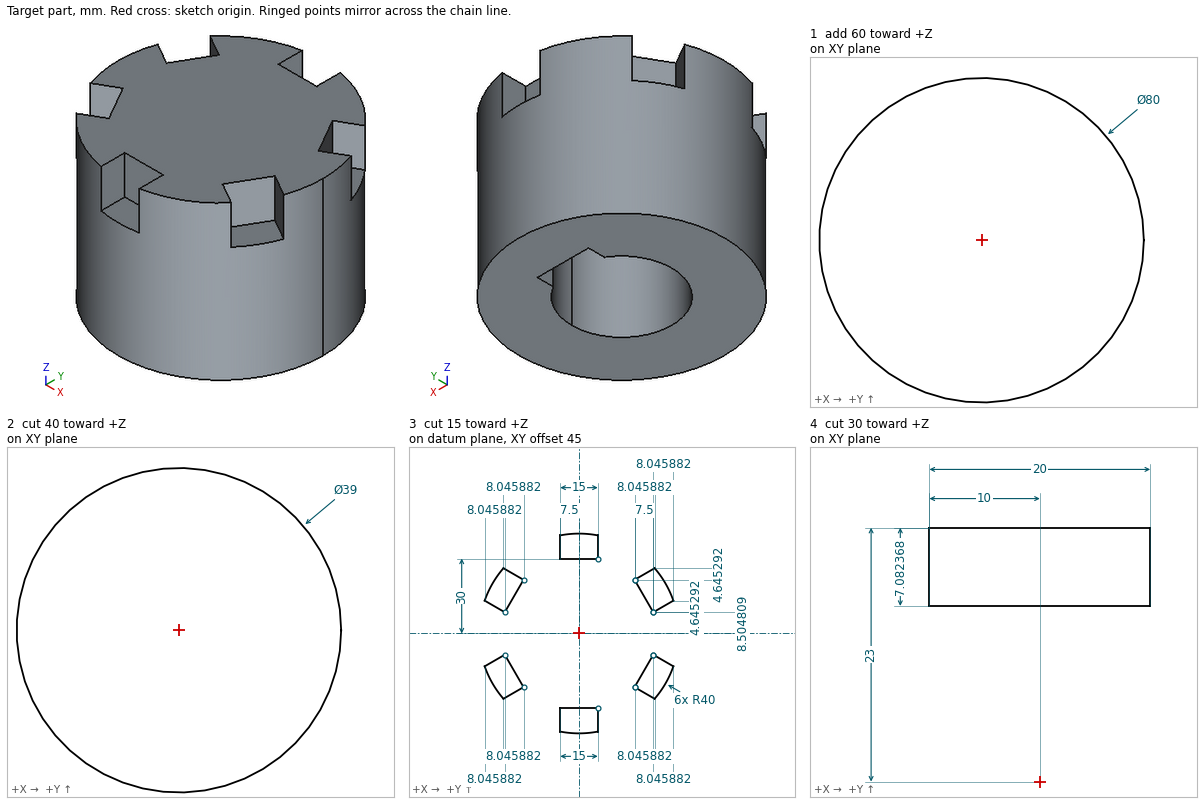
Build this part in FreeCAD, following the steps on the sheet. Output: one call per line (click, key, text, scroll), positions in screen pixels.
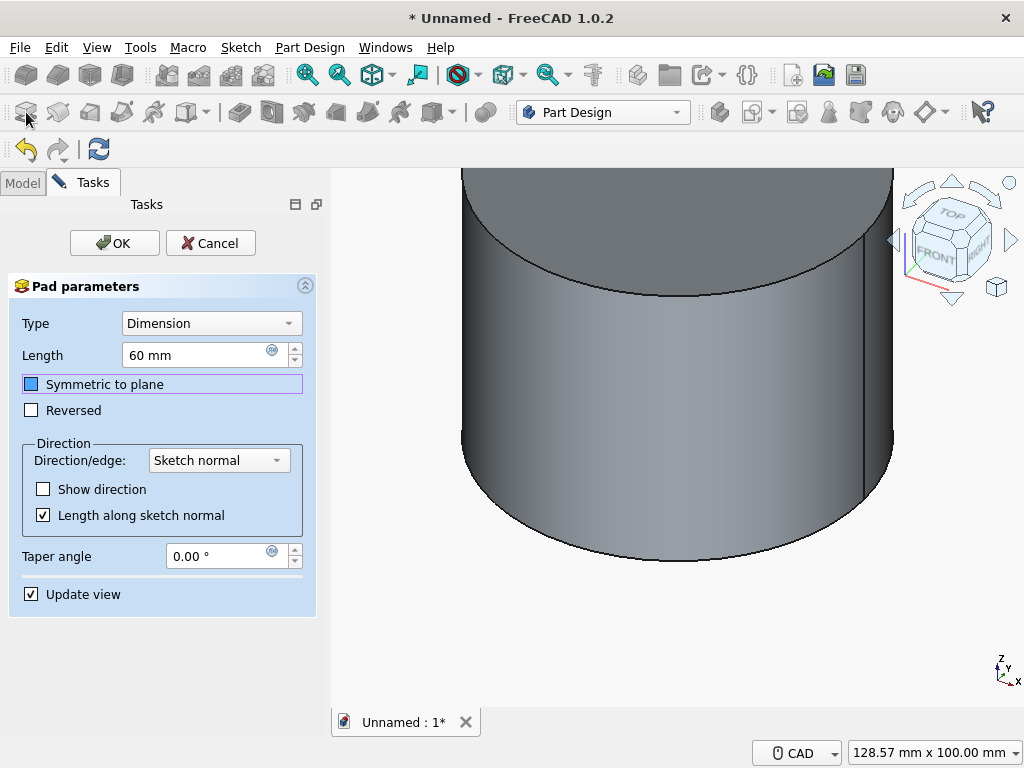
click(115, 243)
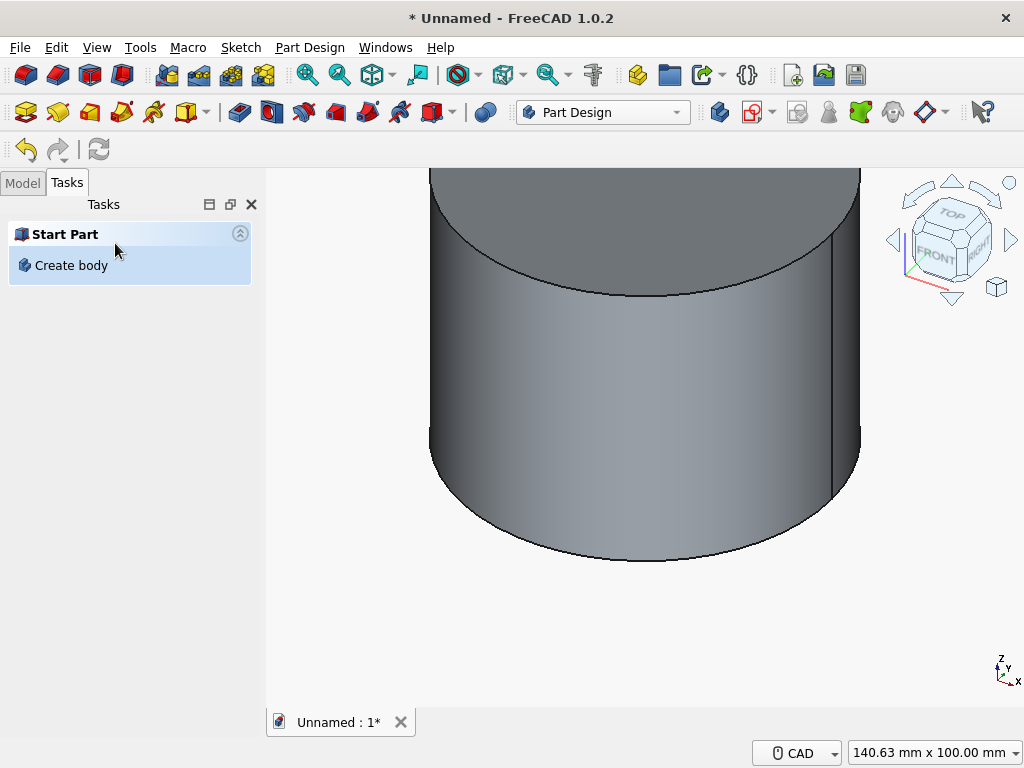
click(308, 76)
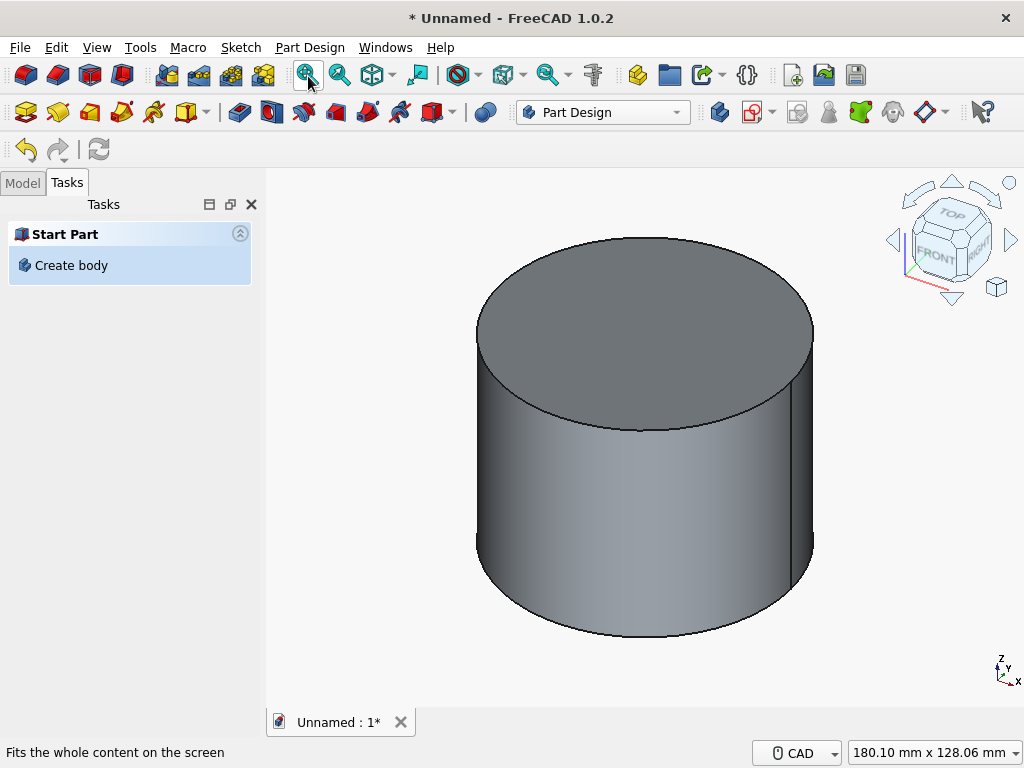
click(752, 112)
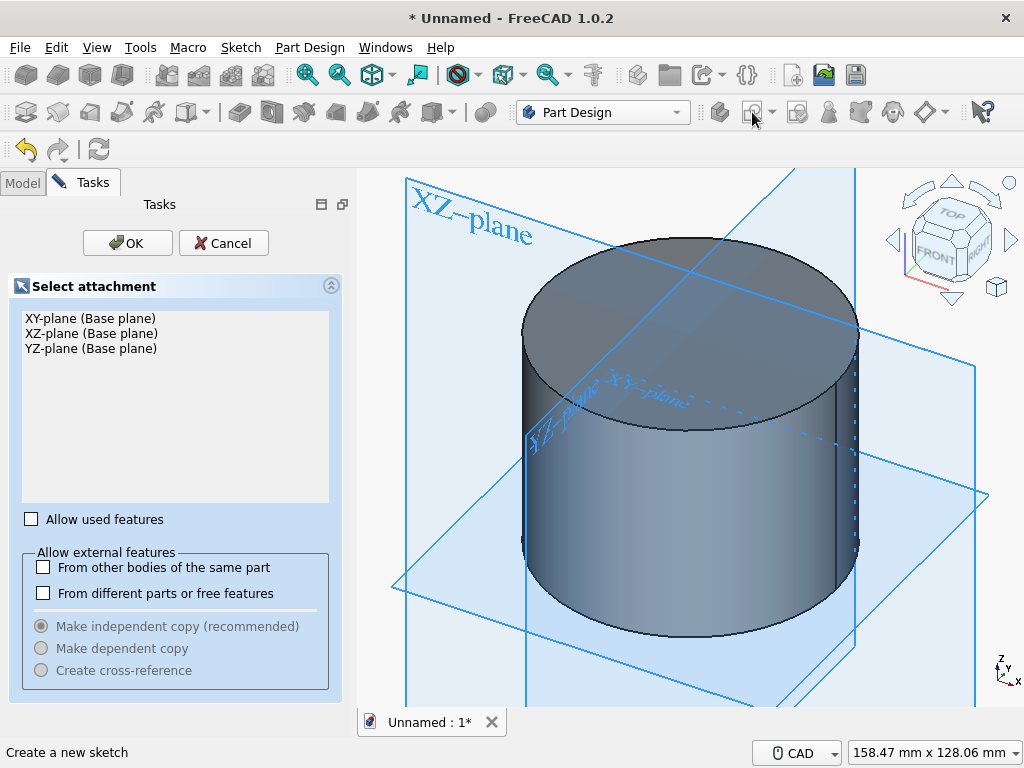
click(82, 318)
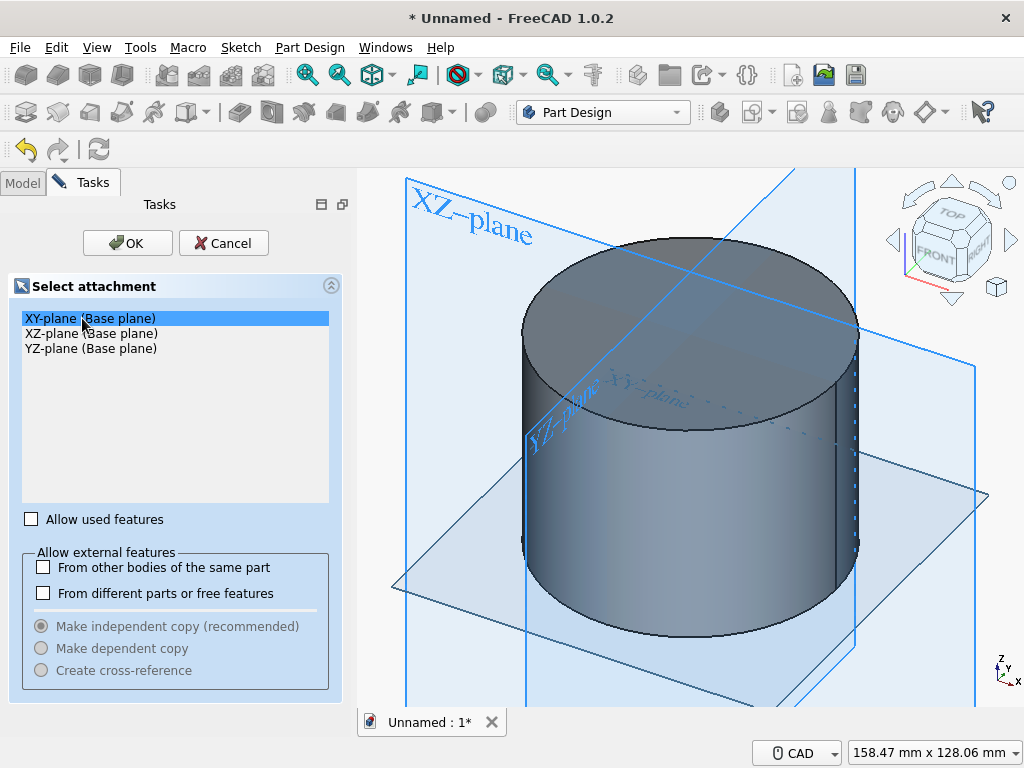
click(128, 243)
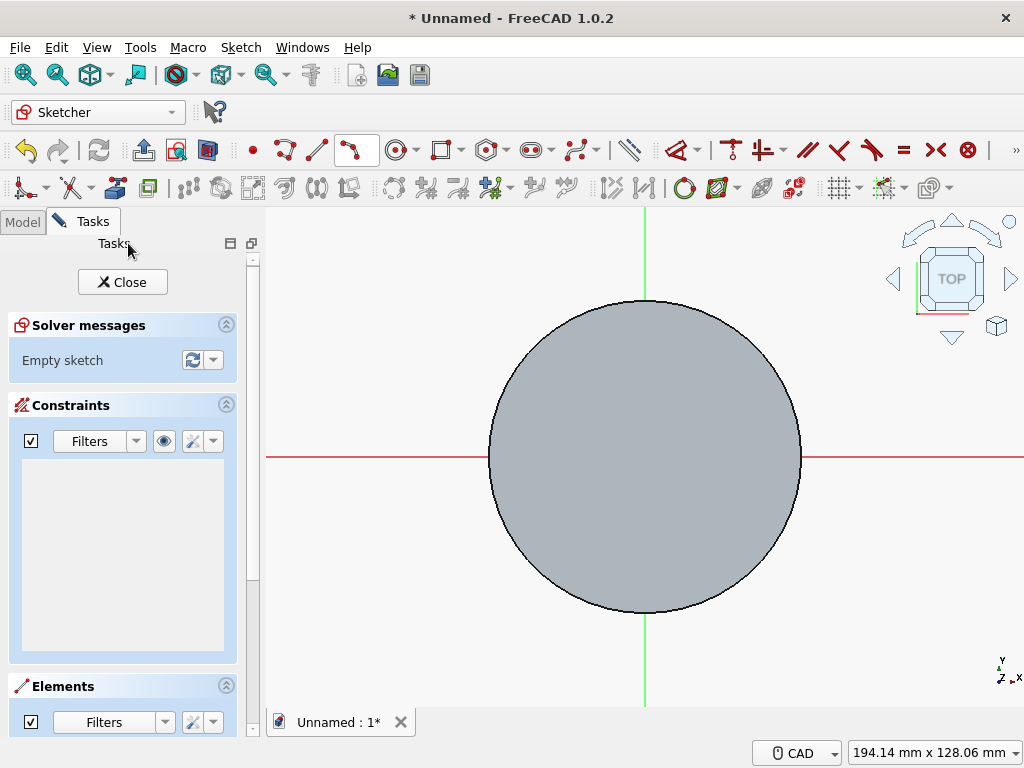
click(208, 150)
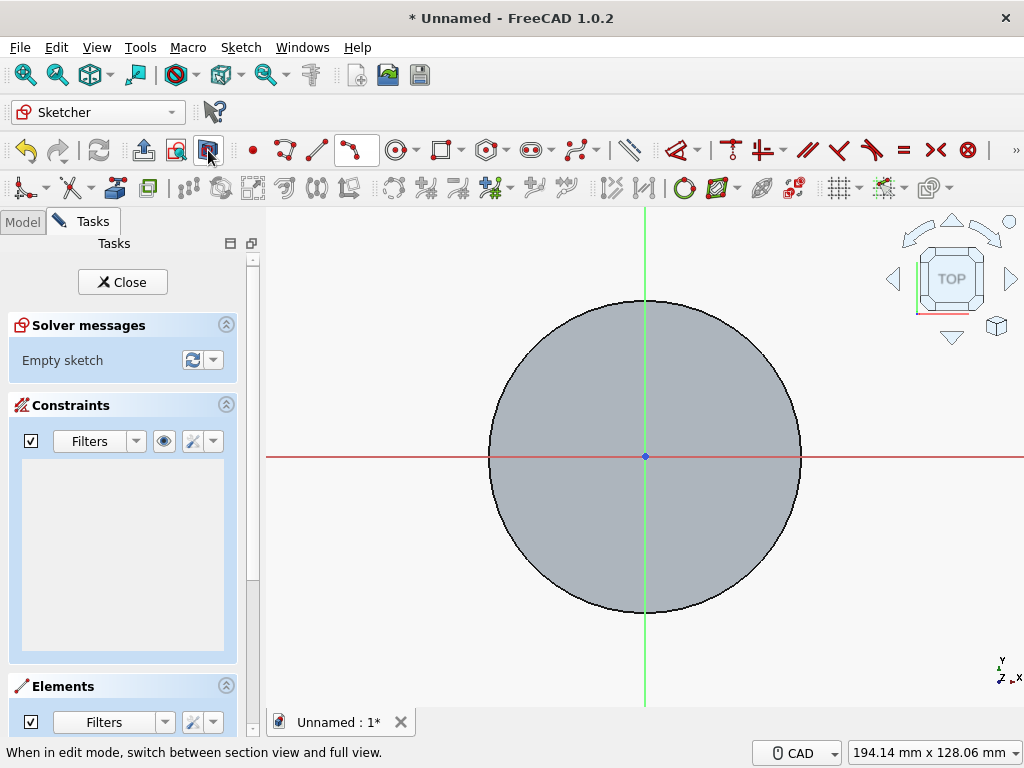
scroll(701, 457, up, 4)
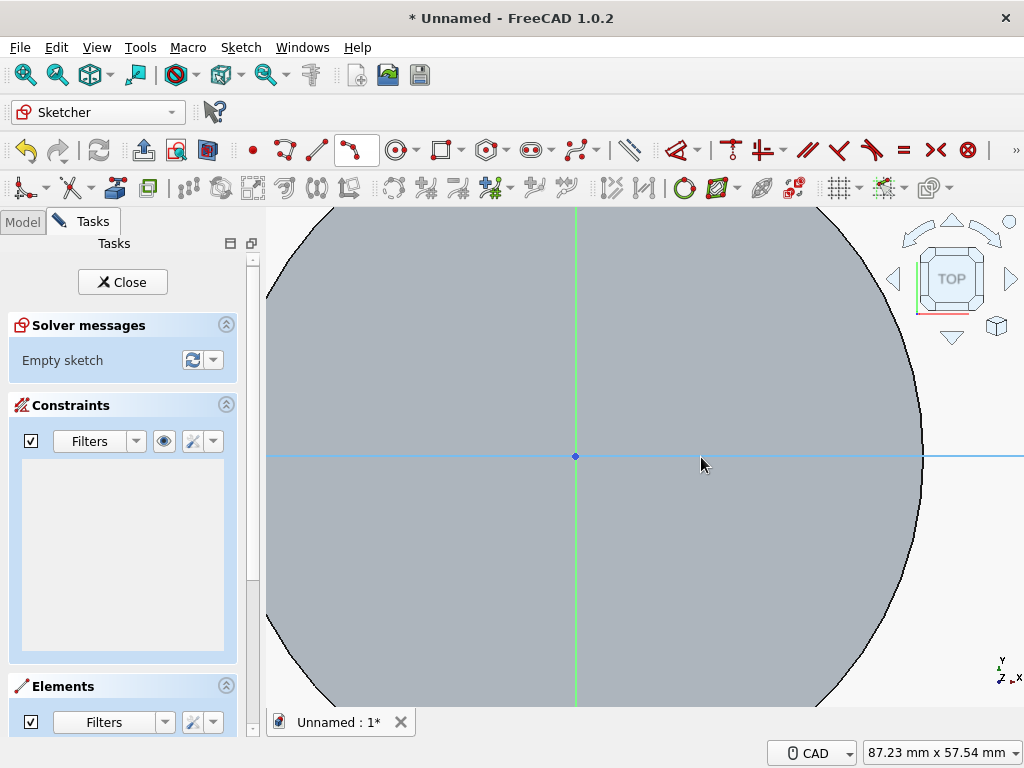
click(396, 150)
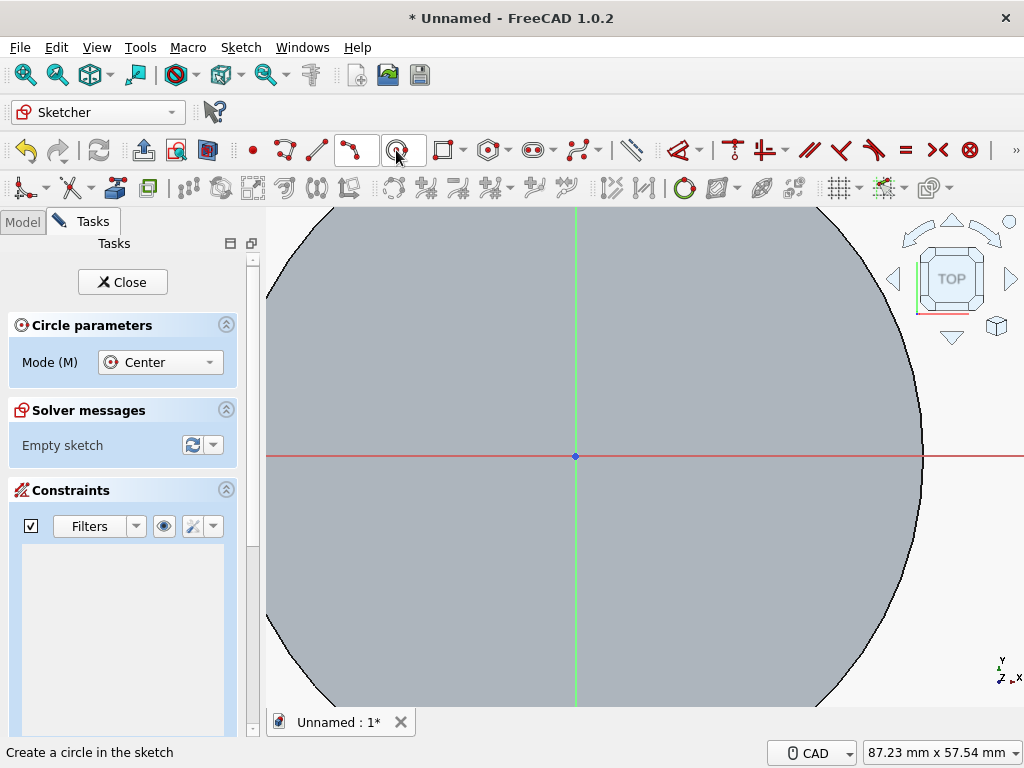
click(576, 456)
click(695, 337)
key(Escape)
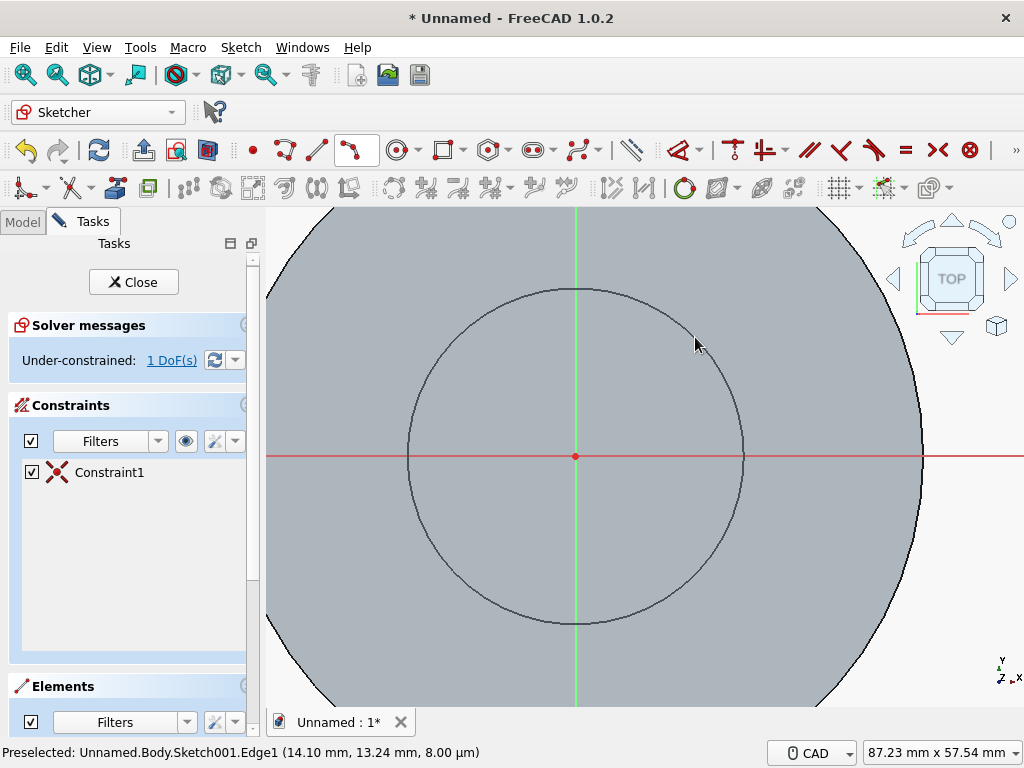
click(678, 150)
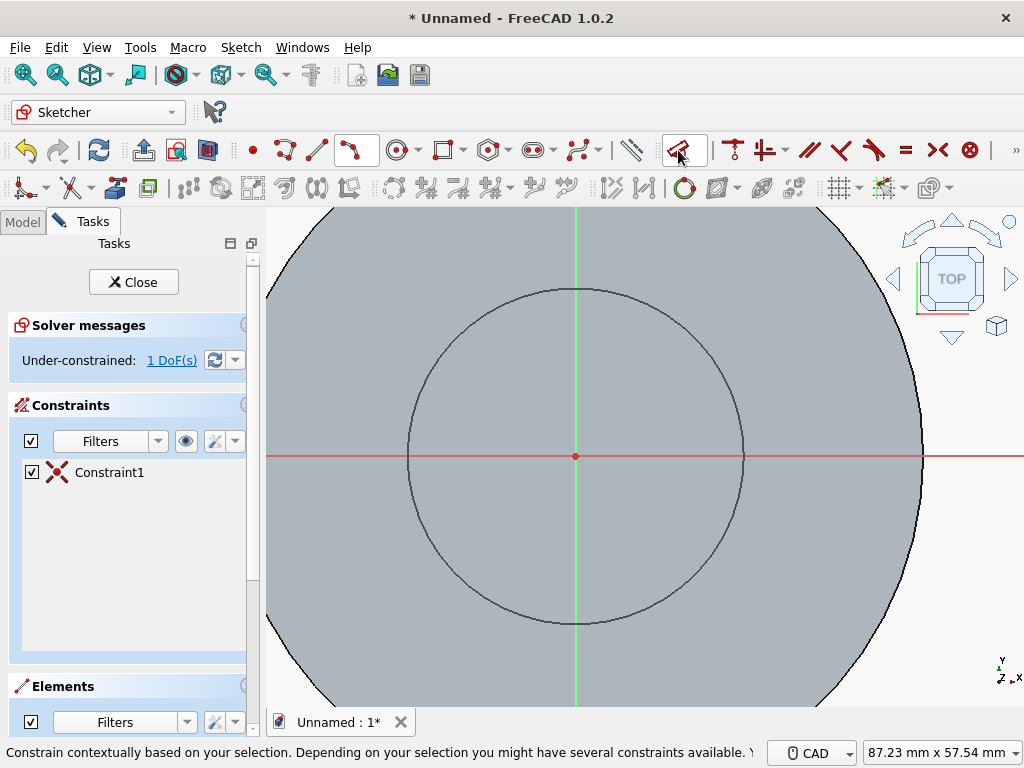
click(694, 337)
click(717, 314)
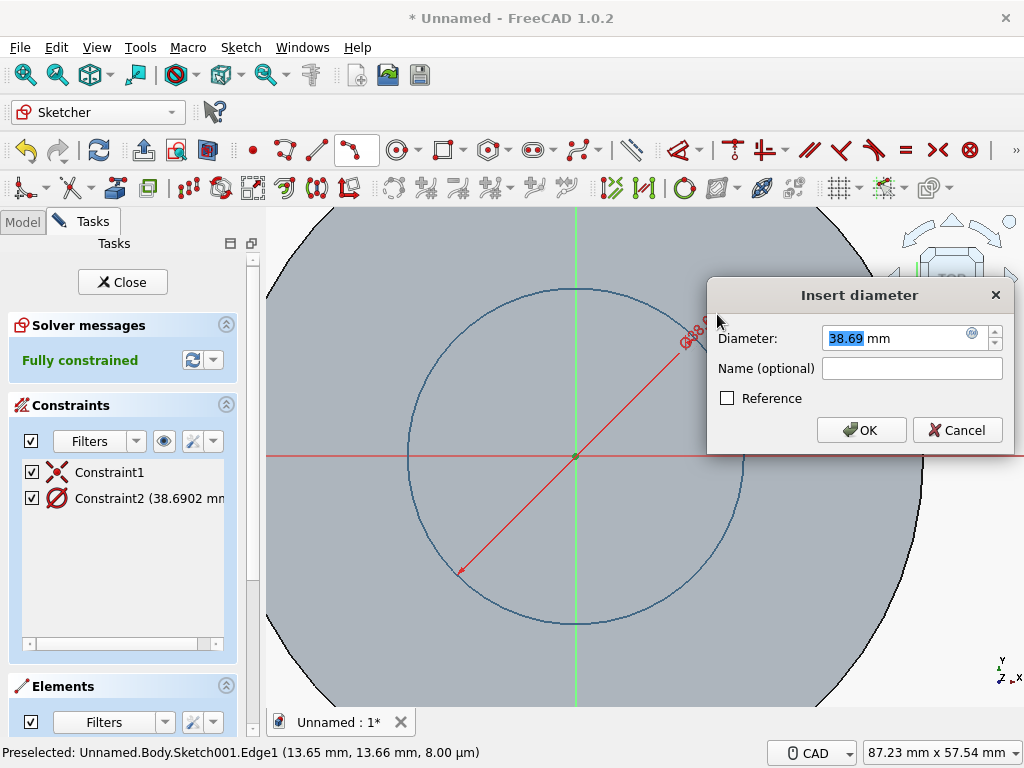
text(39)
key(Return)
key(Escape)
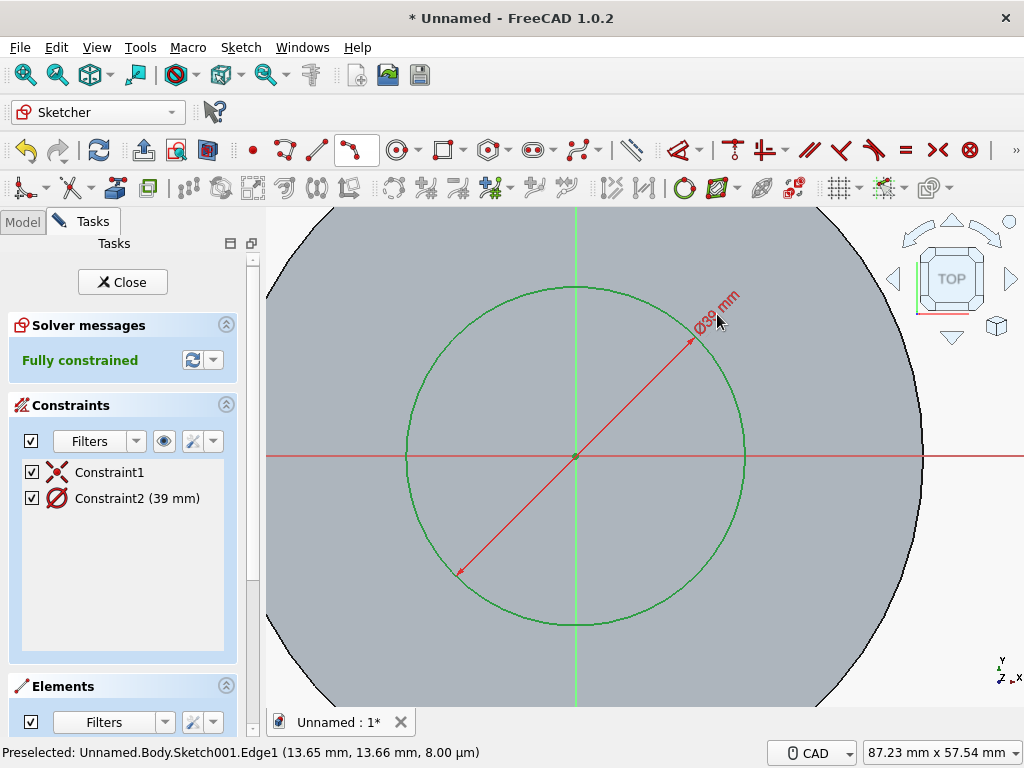
click(123, 282)